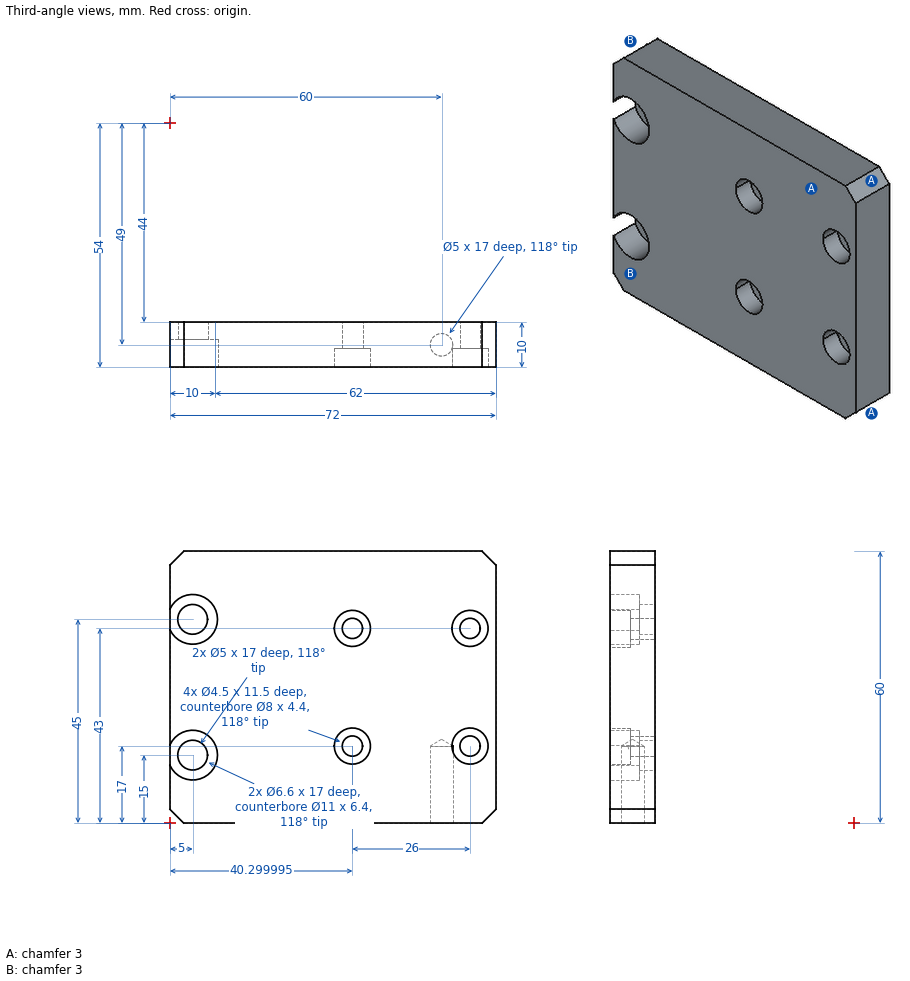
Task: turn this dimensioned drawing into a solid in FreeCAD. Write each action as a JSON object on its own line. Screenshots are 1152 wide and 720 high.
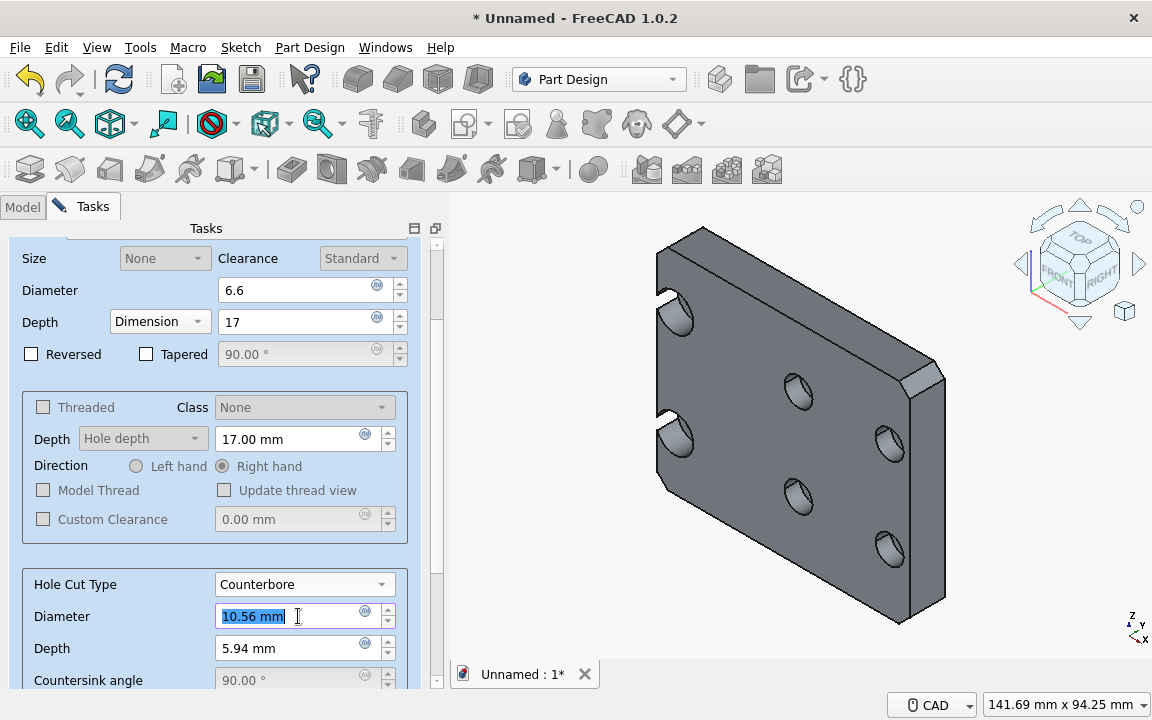
{"action": "type", "text": "11"}
{"action": "key", "text": "Tab"}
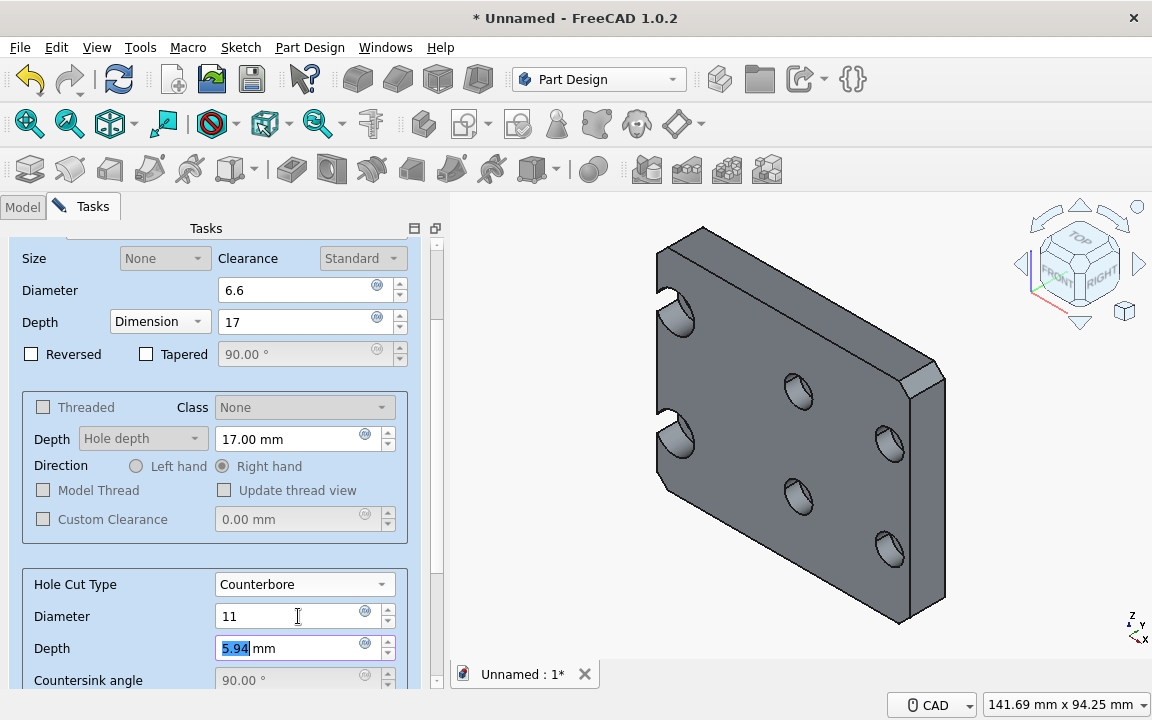
{"action": "type", "text": "6.4"}
{"action": "key", "text": "Tab"}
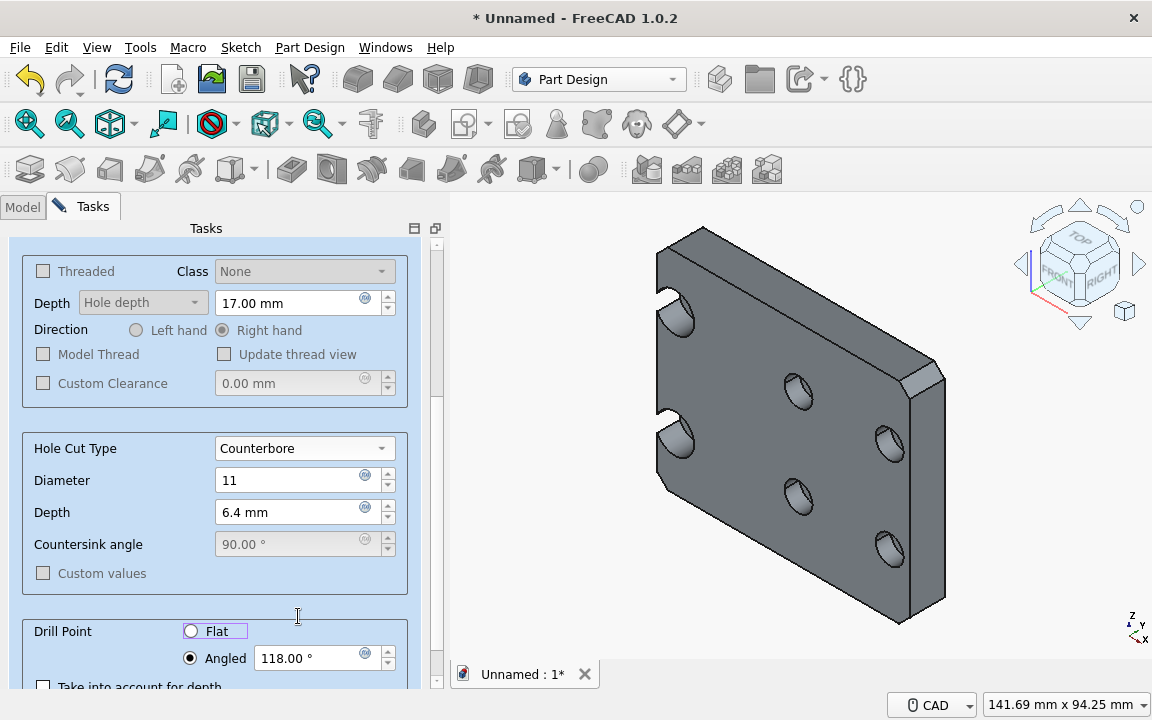
{"action": "scroll", "coordinate": [437, 463], "scroll_direction": "up", "scroll_amount": 6}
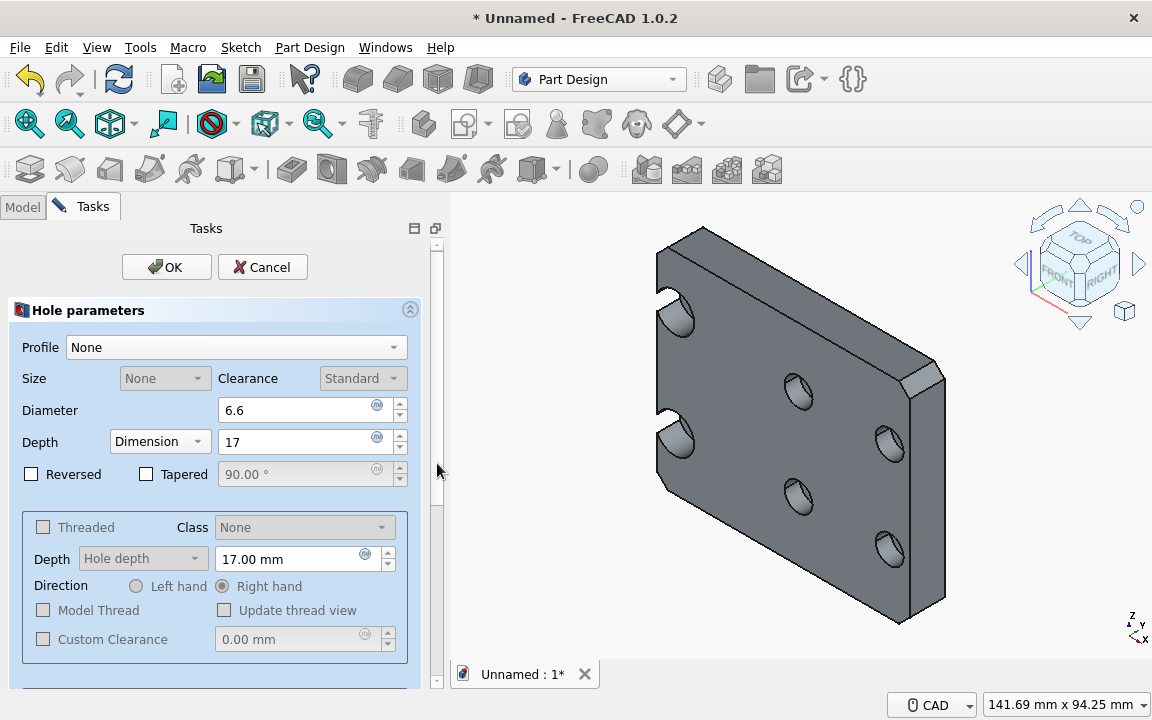
{"action": "left_click", "coordinate": [167, 267]}